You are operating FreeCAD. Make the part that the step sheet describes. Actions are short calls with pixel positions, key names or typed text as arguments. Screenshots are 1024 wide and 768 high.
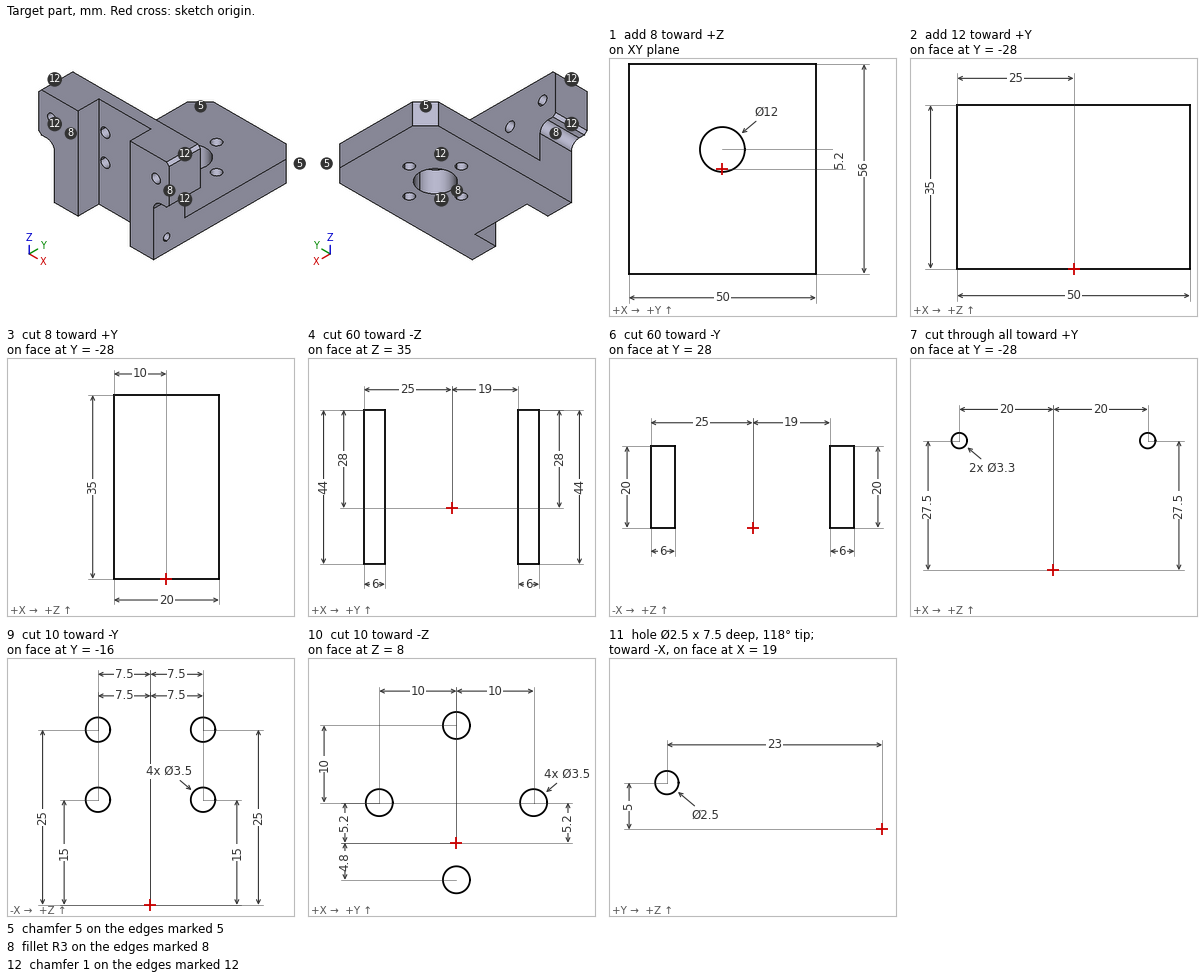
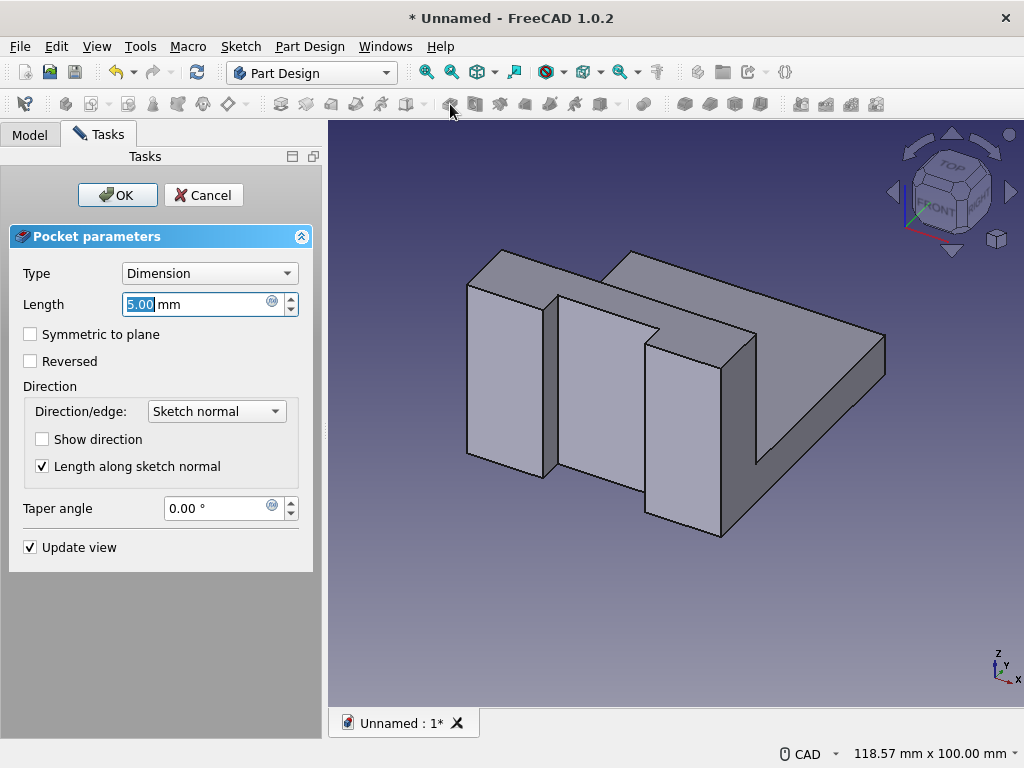
text(8)
key(Tab)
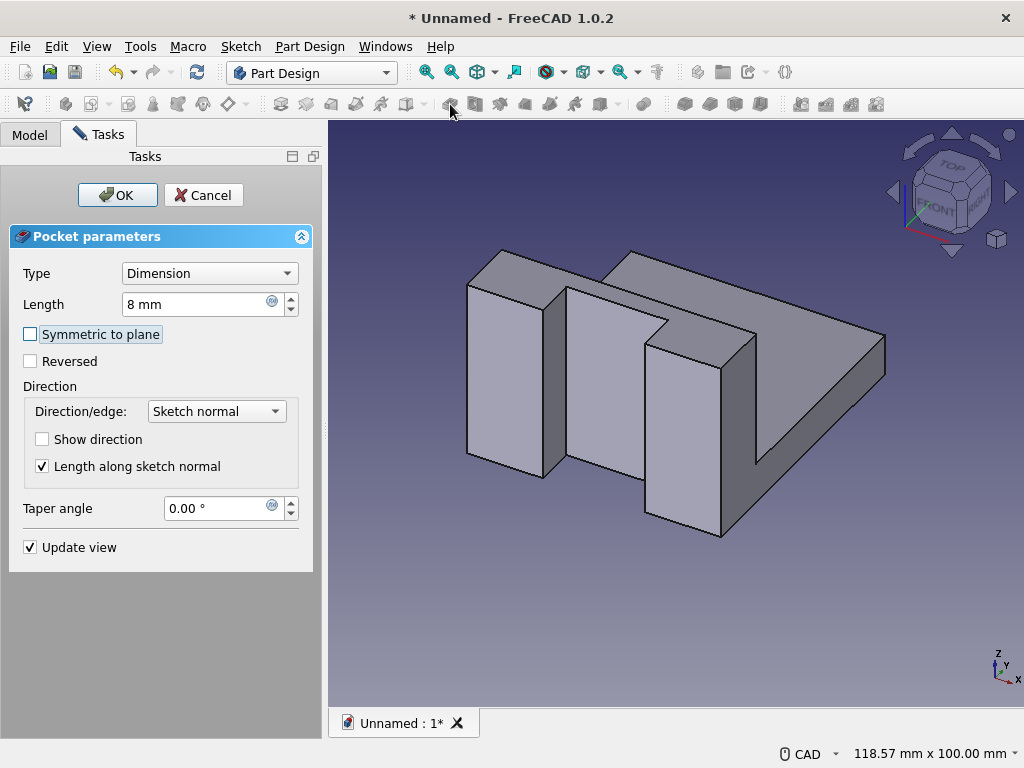
click(118, 195)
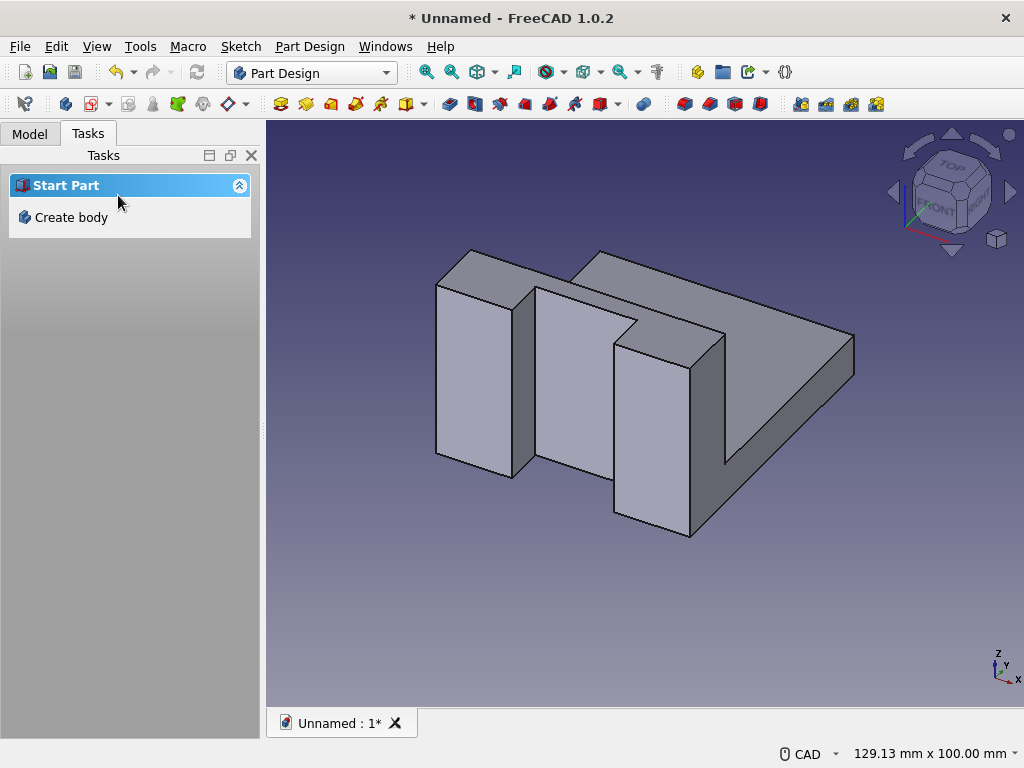
click(653, 332)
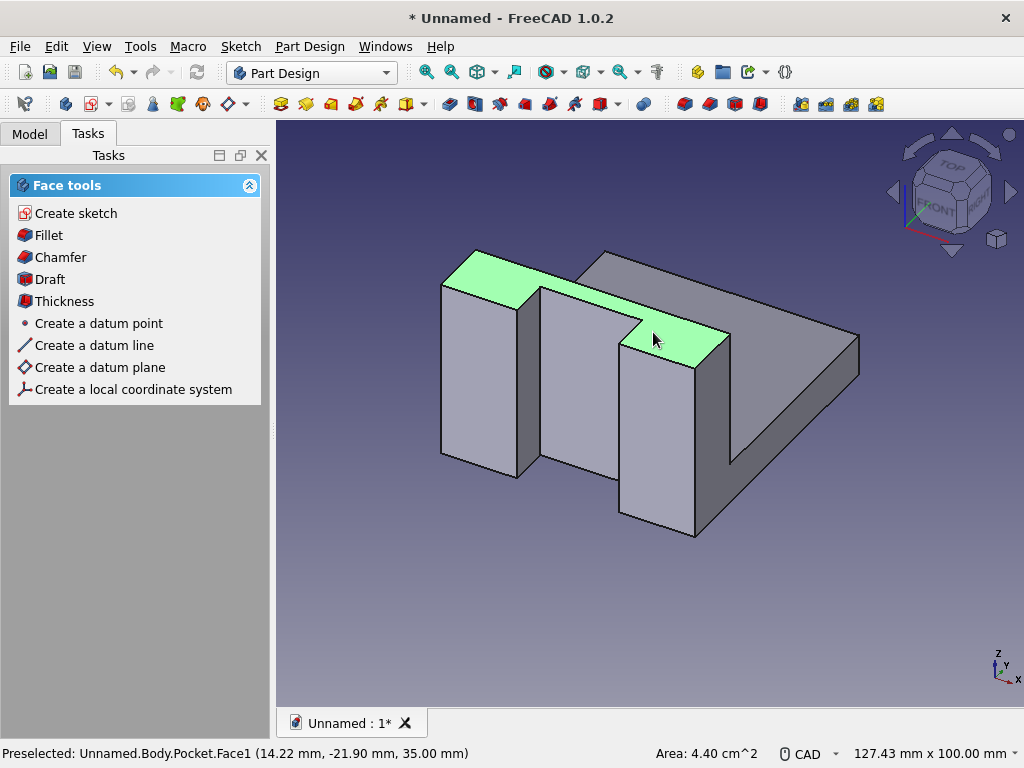
click(90, 104)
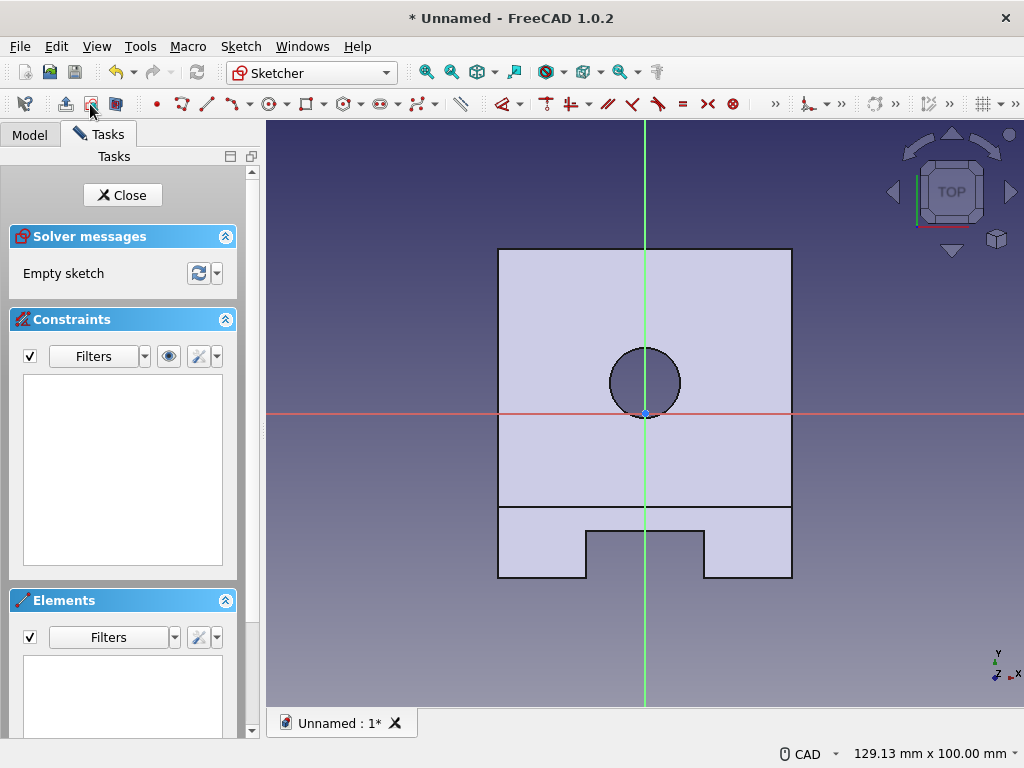
scroll(784, 307, up, 2)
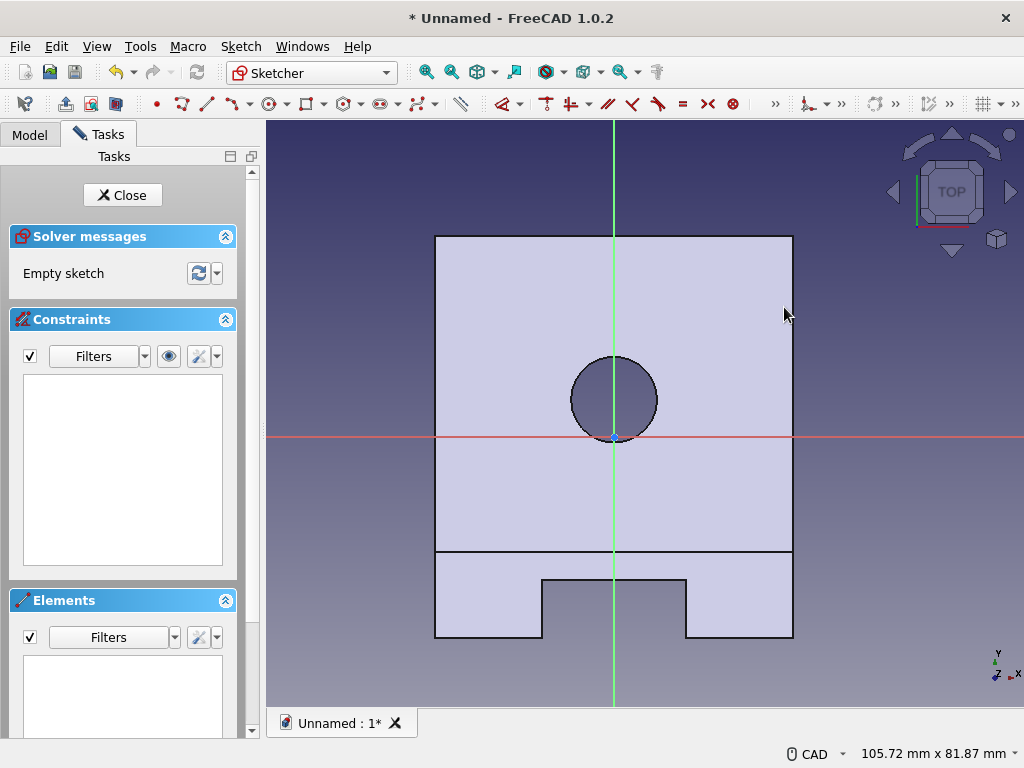
click(306, 104)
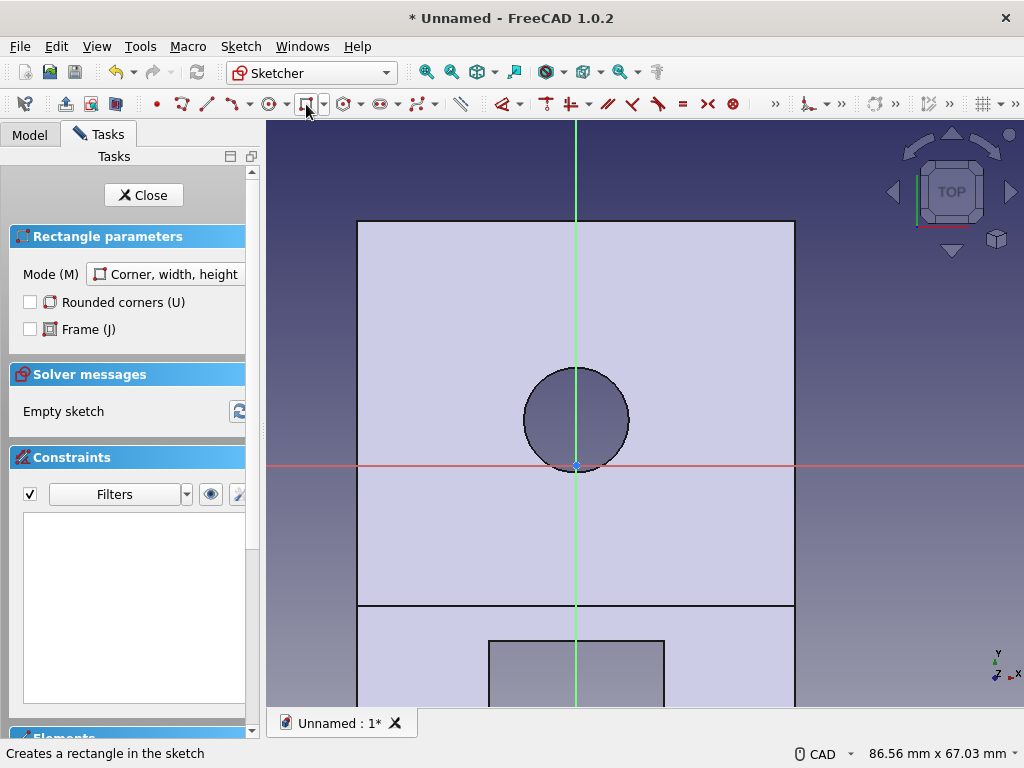
click(357, 221)
move(410, 606)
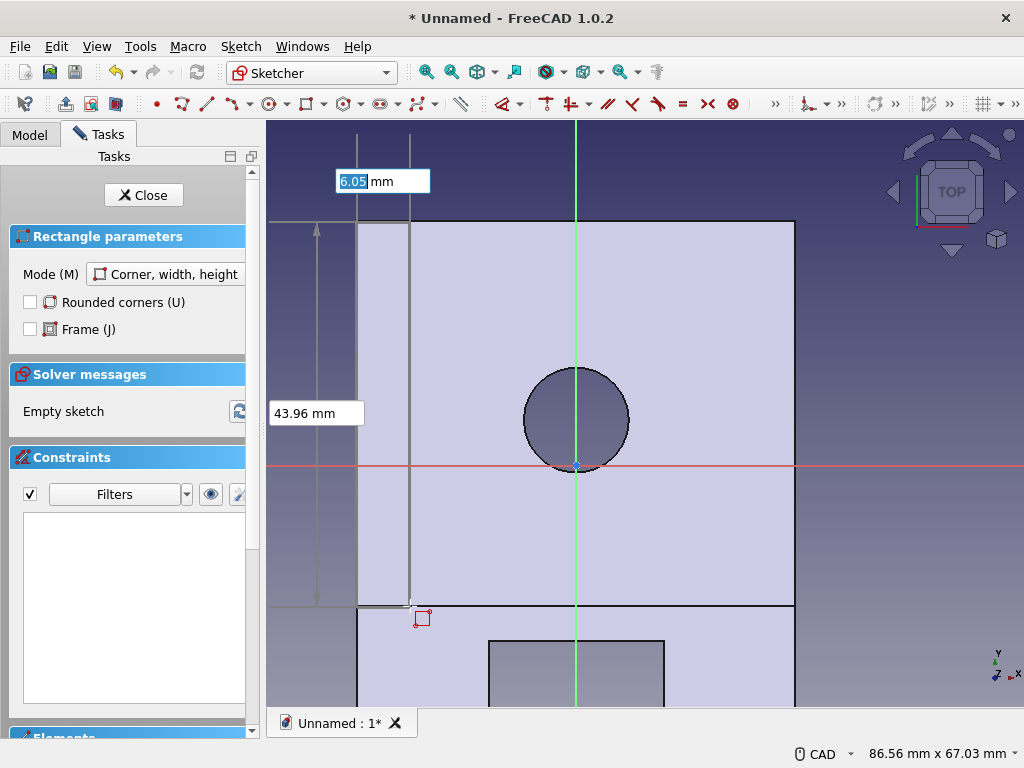
text(6)
key(Tab)
text(44)
key(Return)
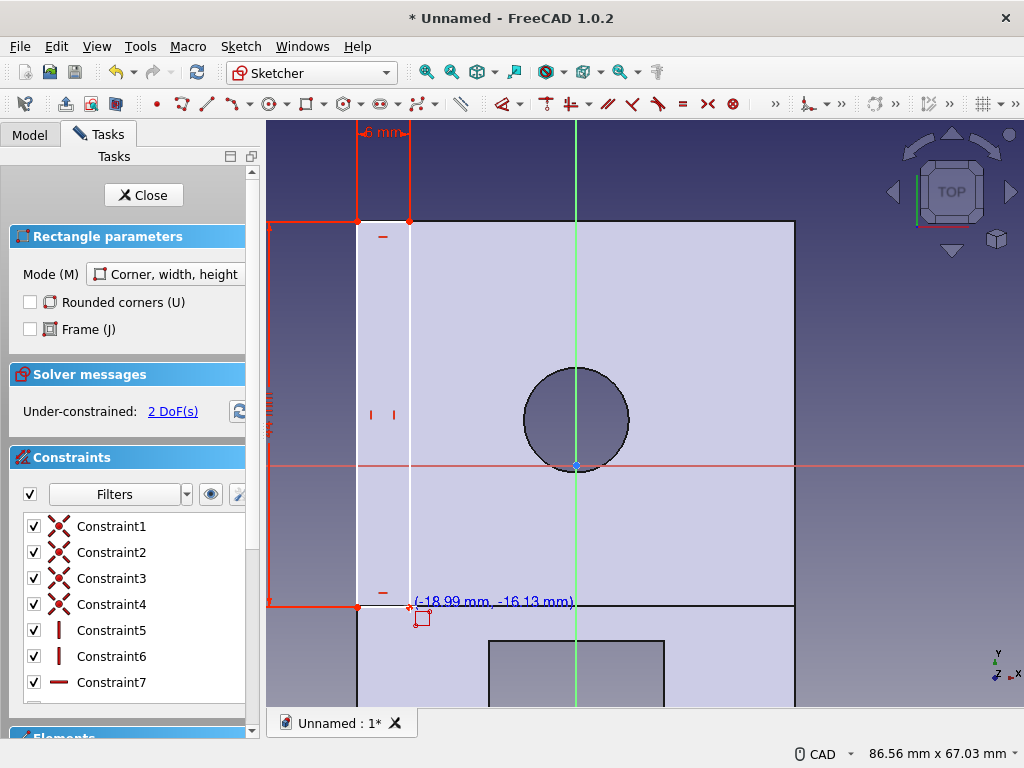
click(743, 221)
move(795, 606)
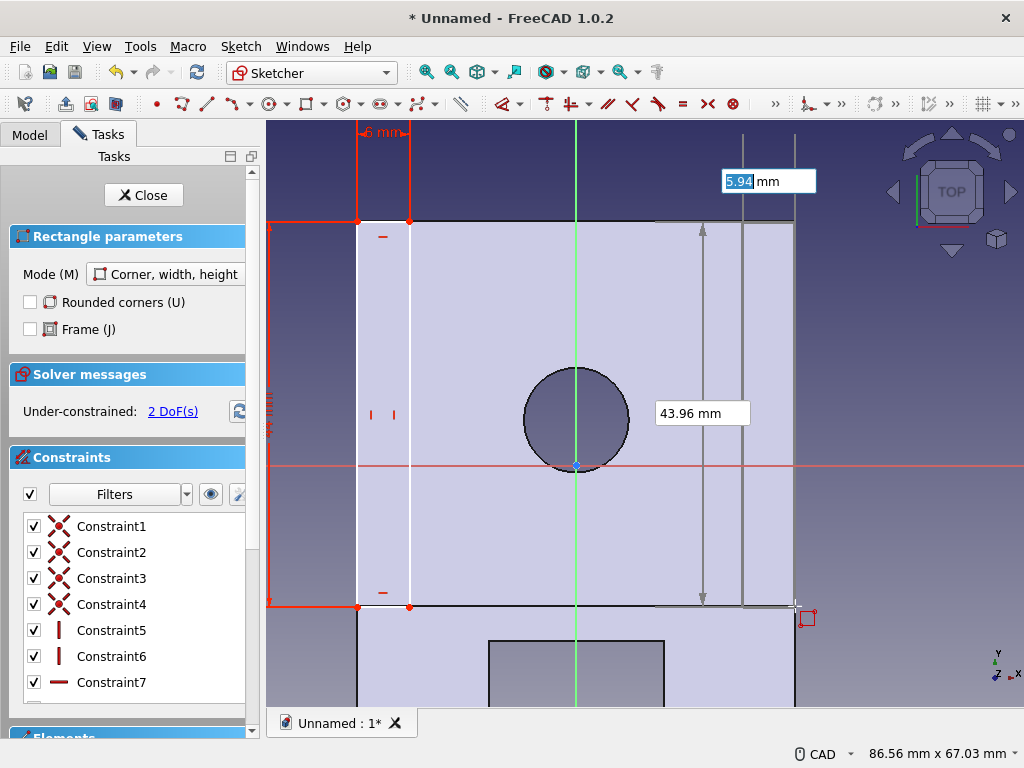
text(6)
key(Tab)
text(44)
key(Return)
key(Escape)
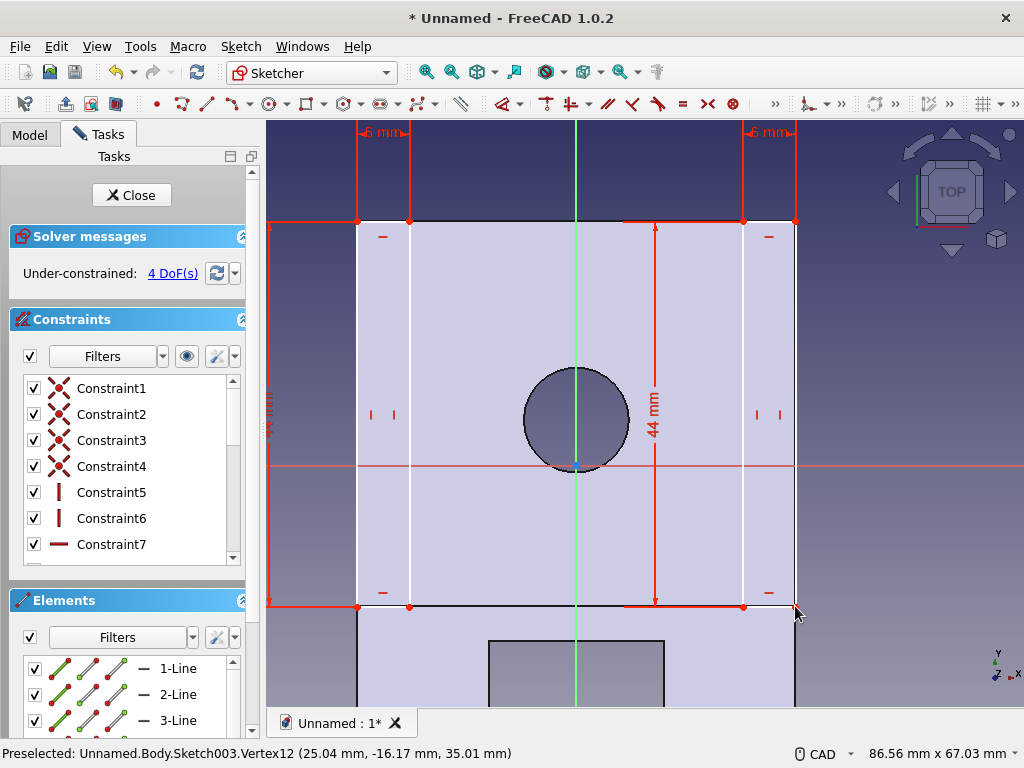
click(502, 104)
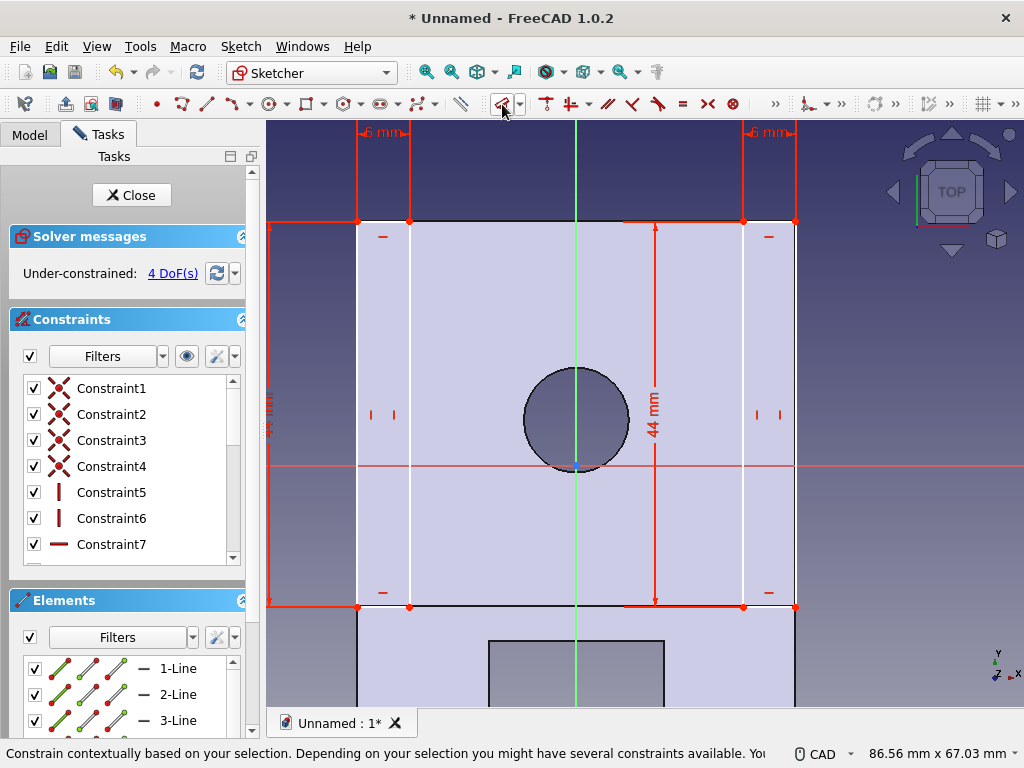
click(357, 222)
click(467, 188)